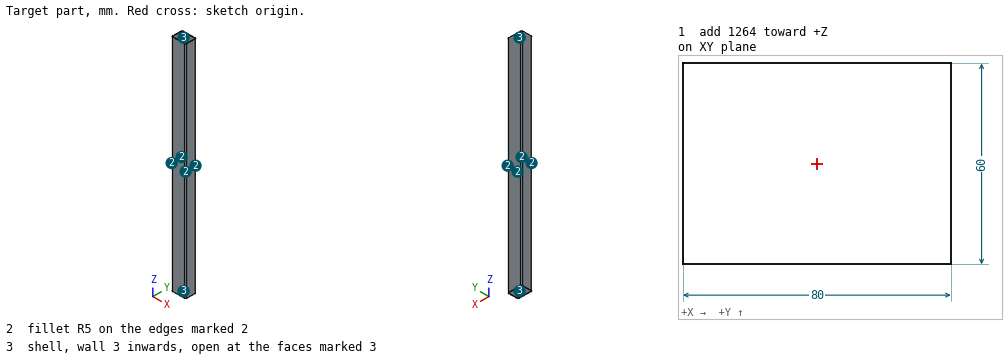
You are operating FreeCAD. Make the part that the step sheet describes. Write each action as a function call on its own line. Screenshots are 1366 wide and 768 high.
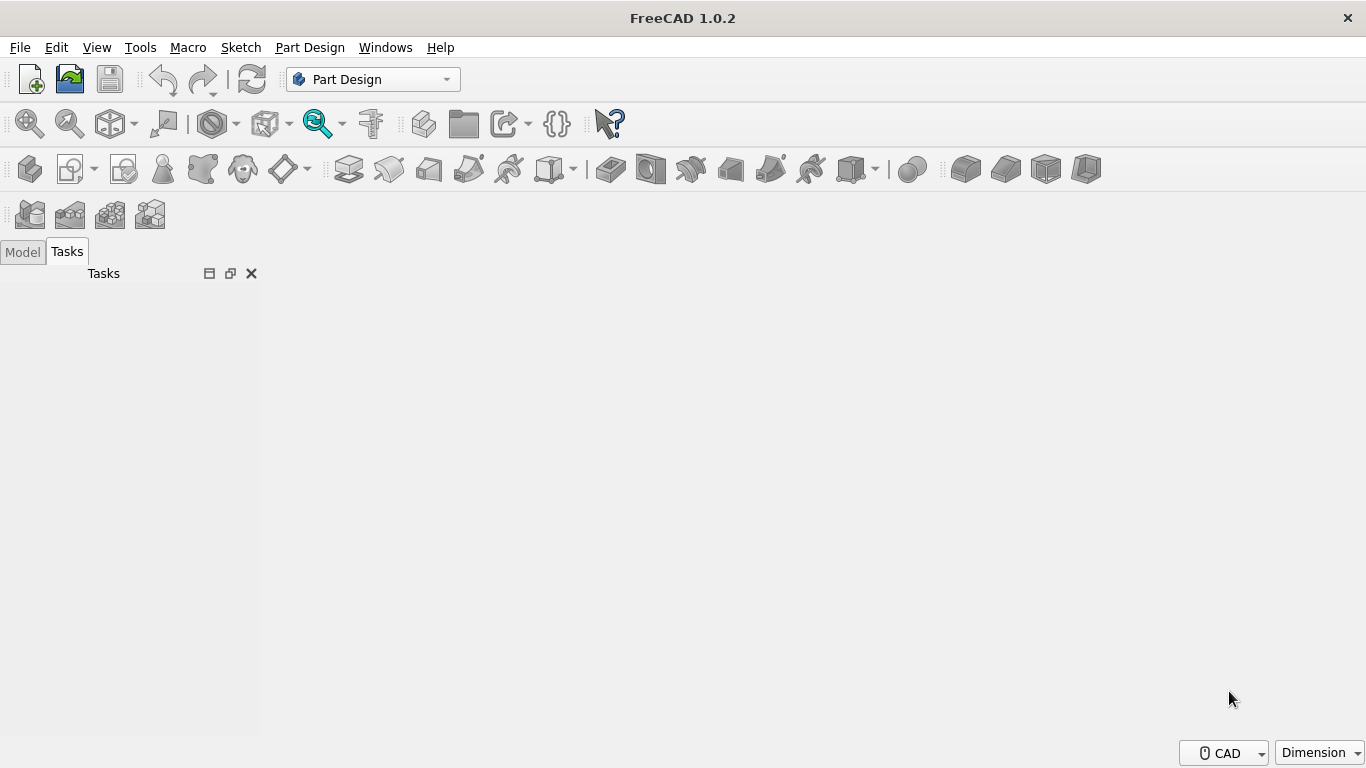
key(ctrl+n)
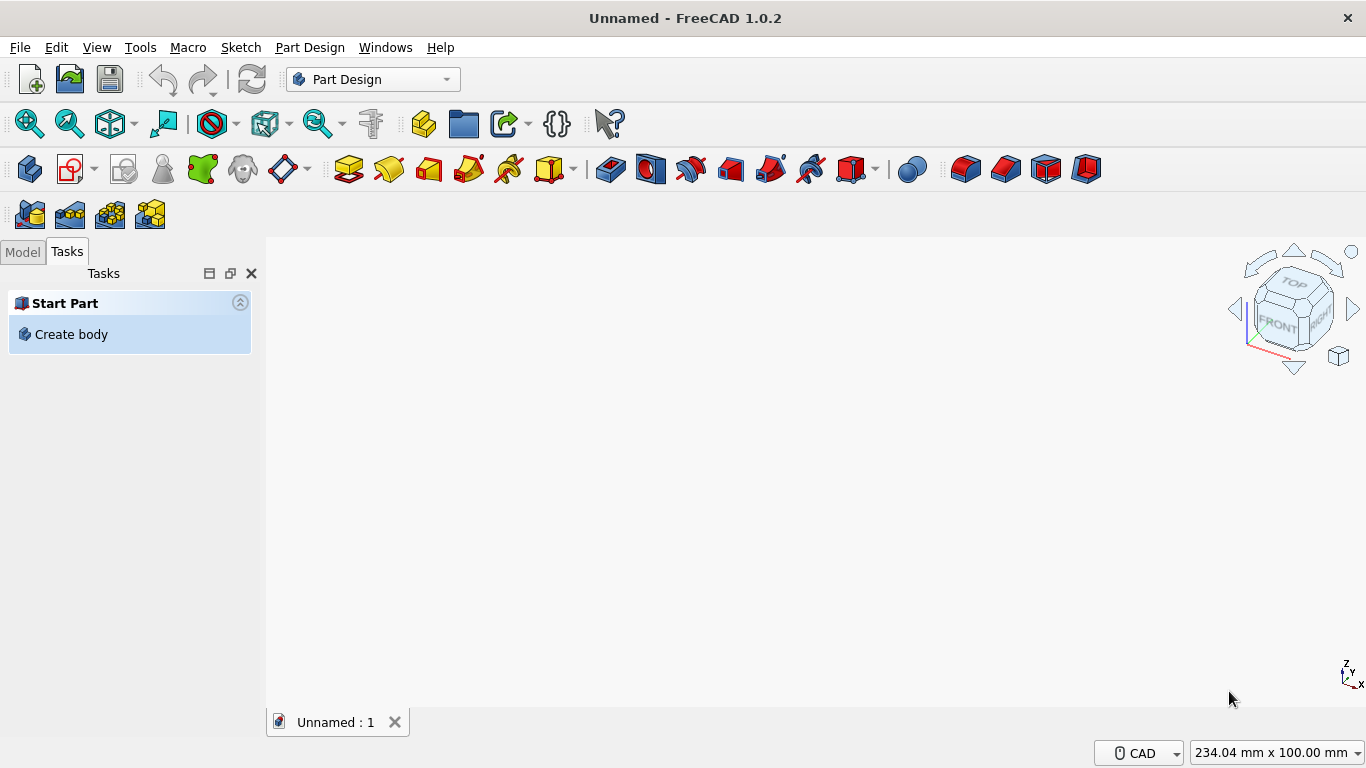
click(70, 170)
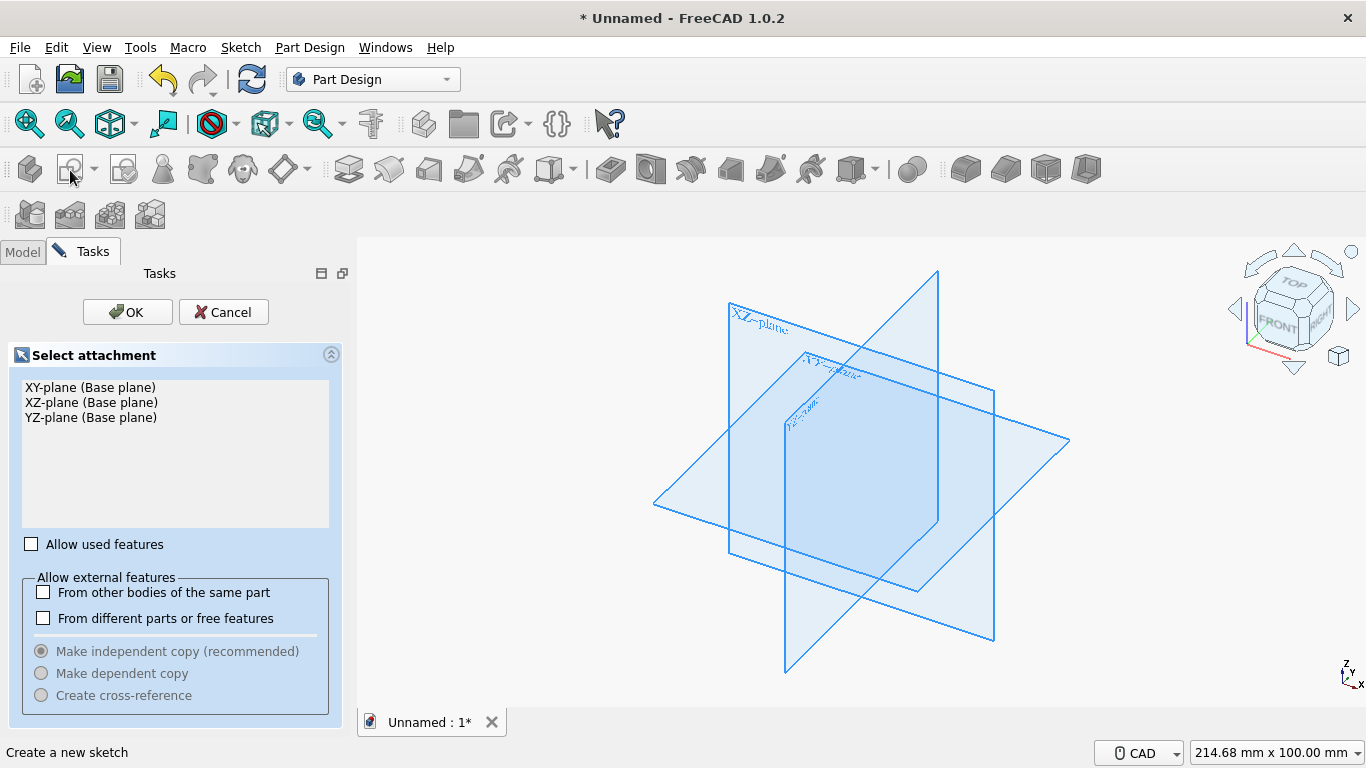
click(82, 388)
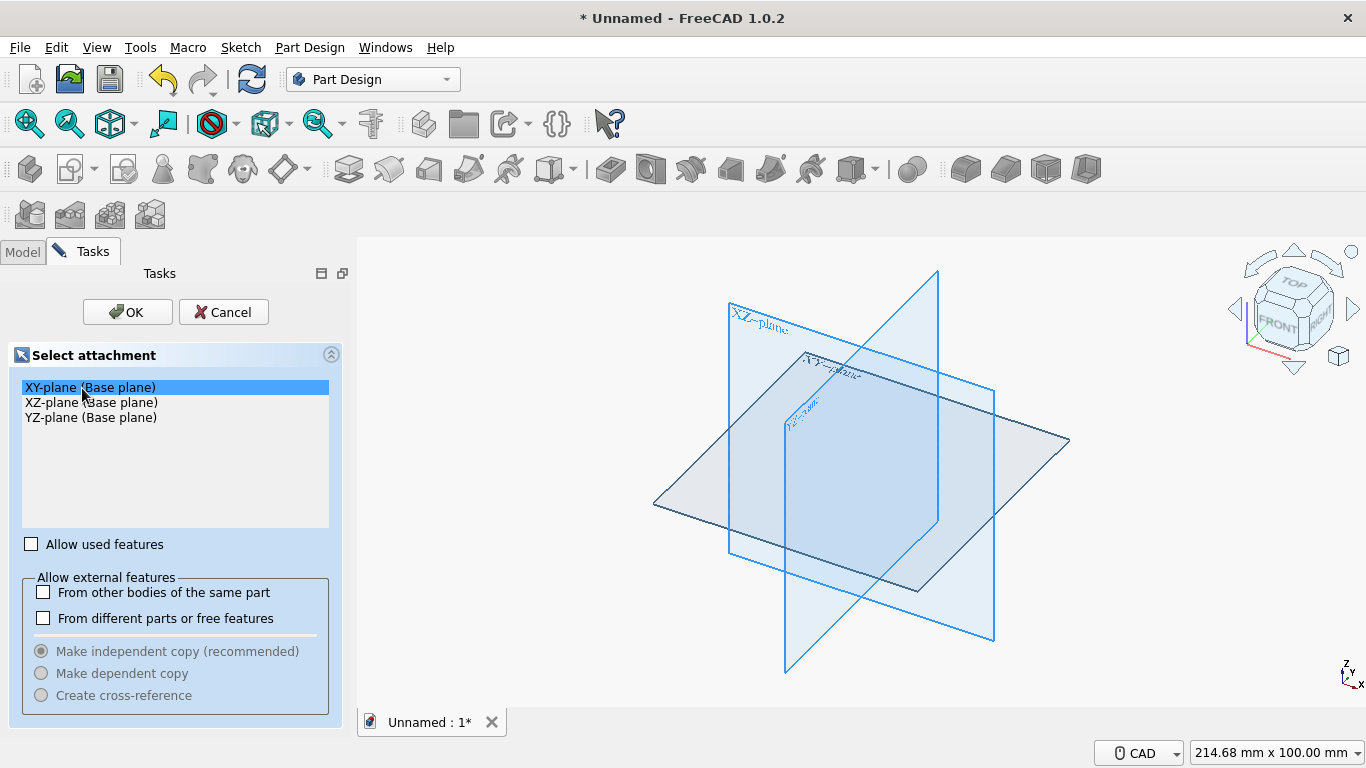
click(128, 312)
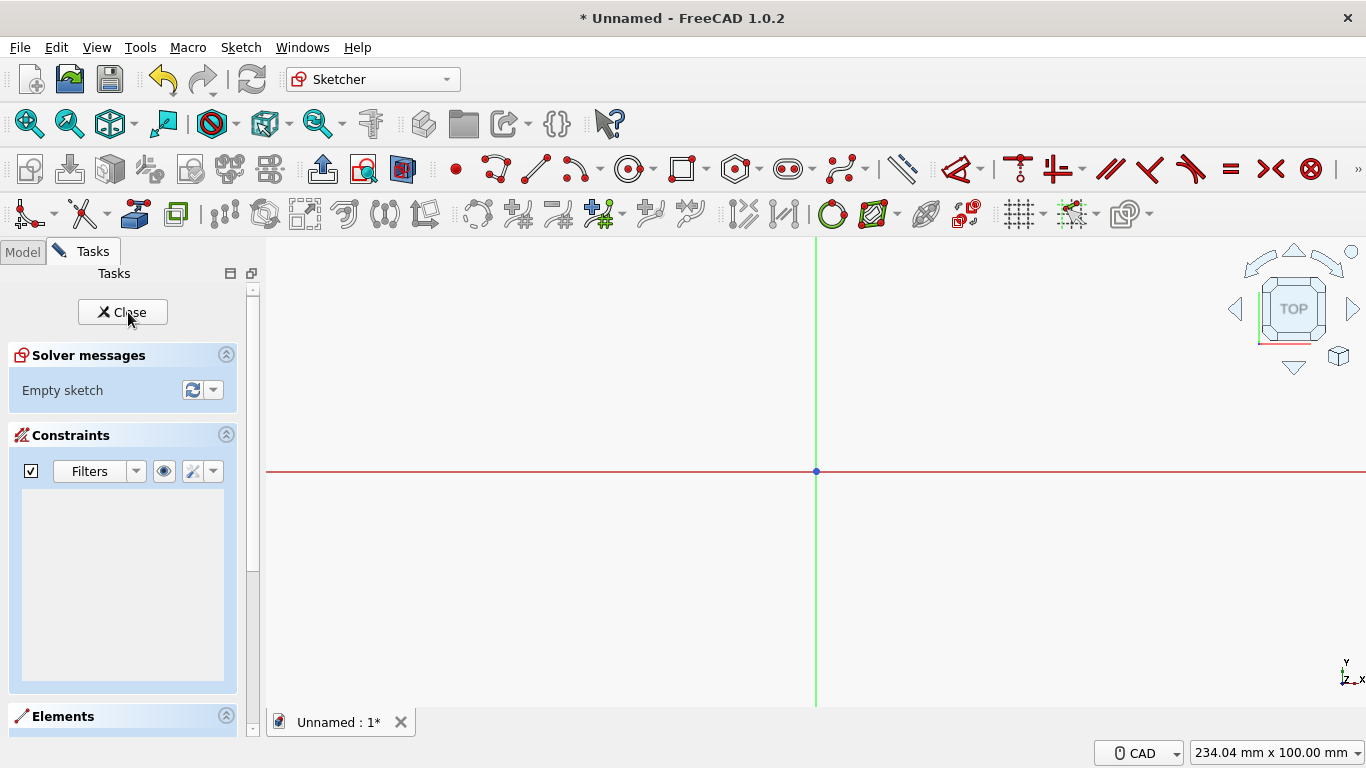
click(708, 170)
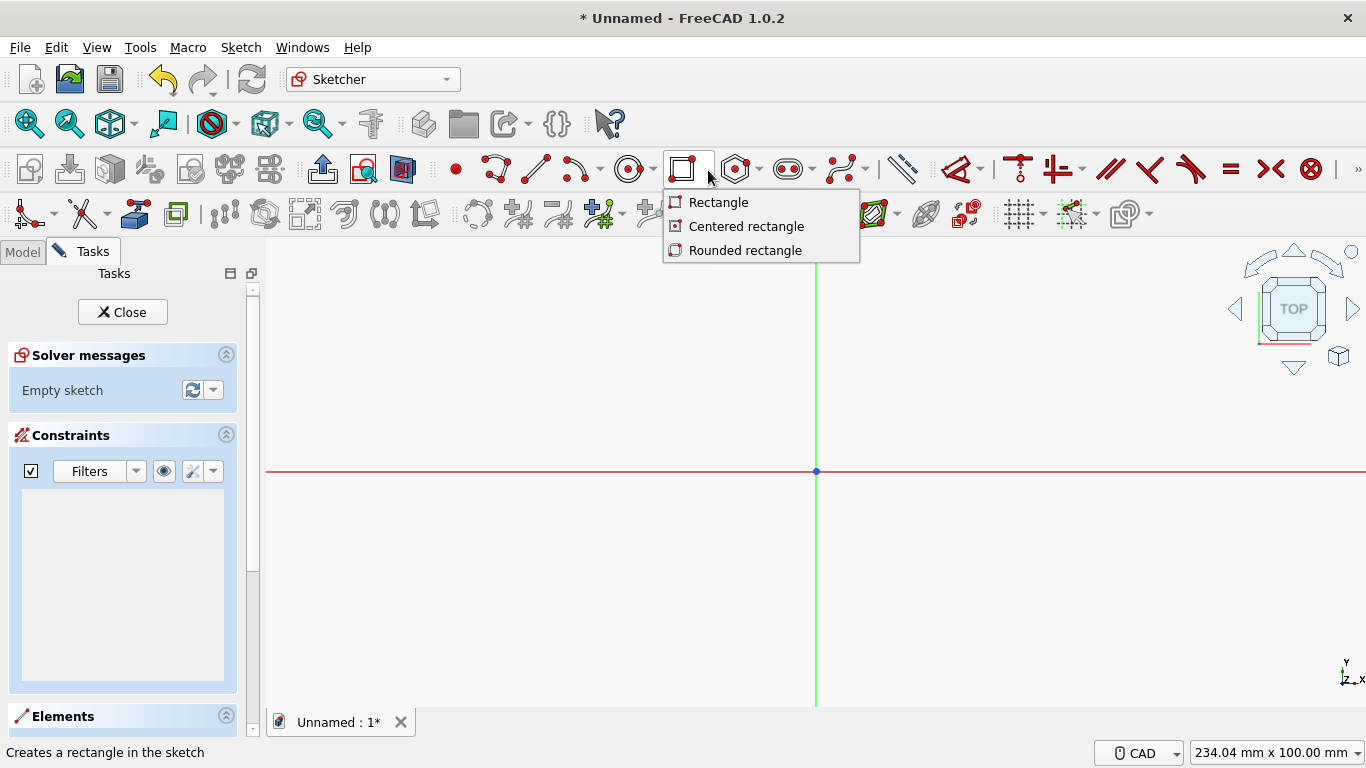
click(762, 226)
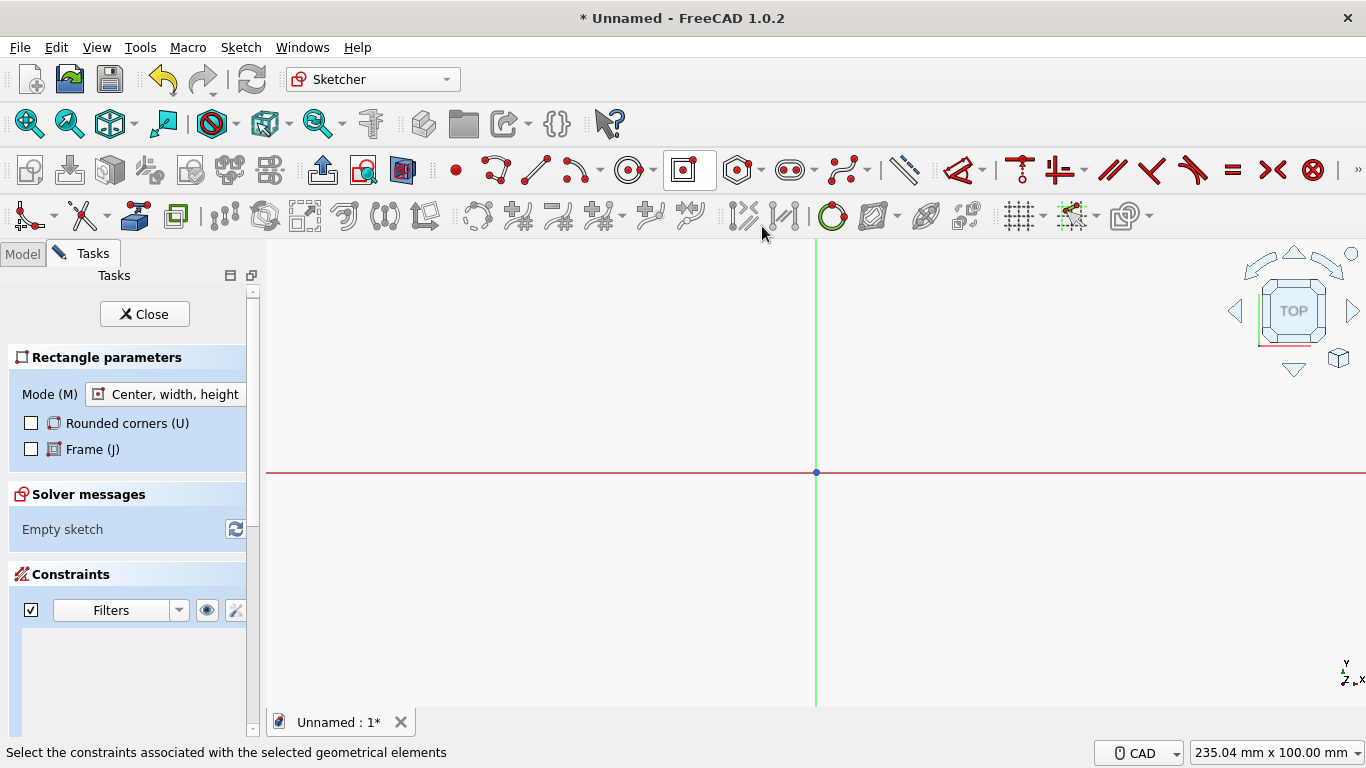
click(816, 473)
move(1003, 333)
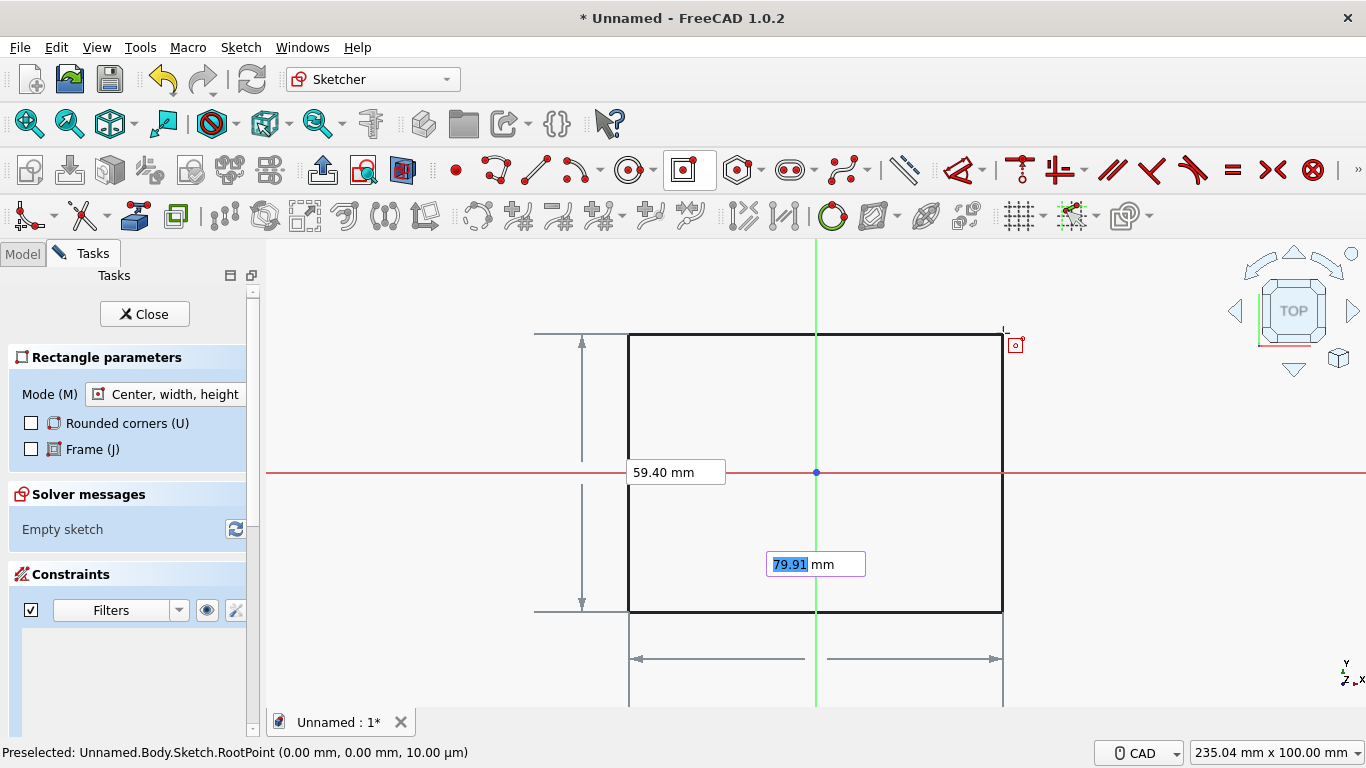
text(80)
key(Tab)
text(60)
key(Return)
key(Escape)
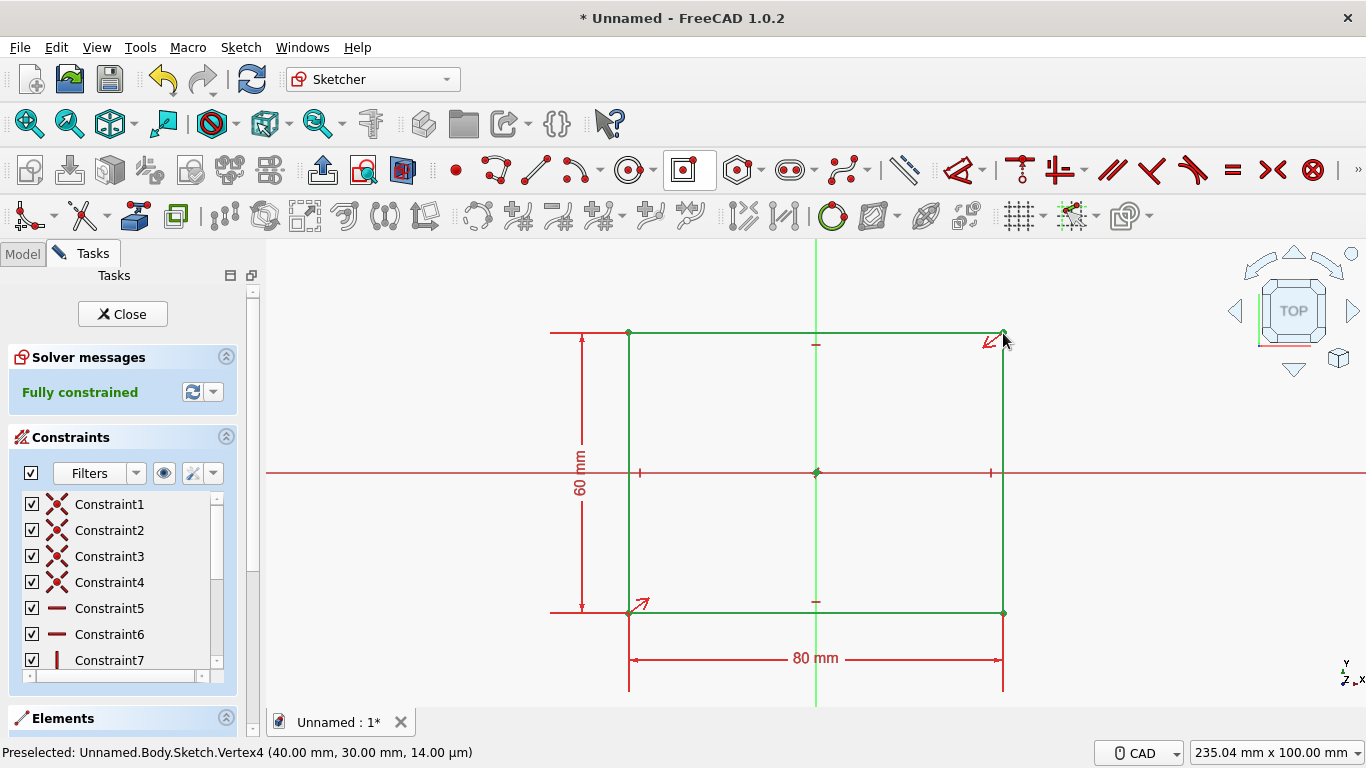
click(123, 314)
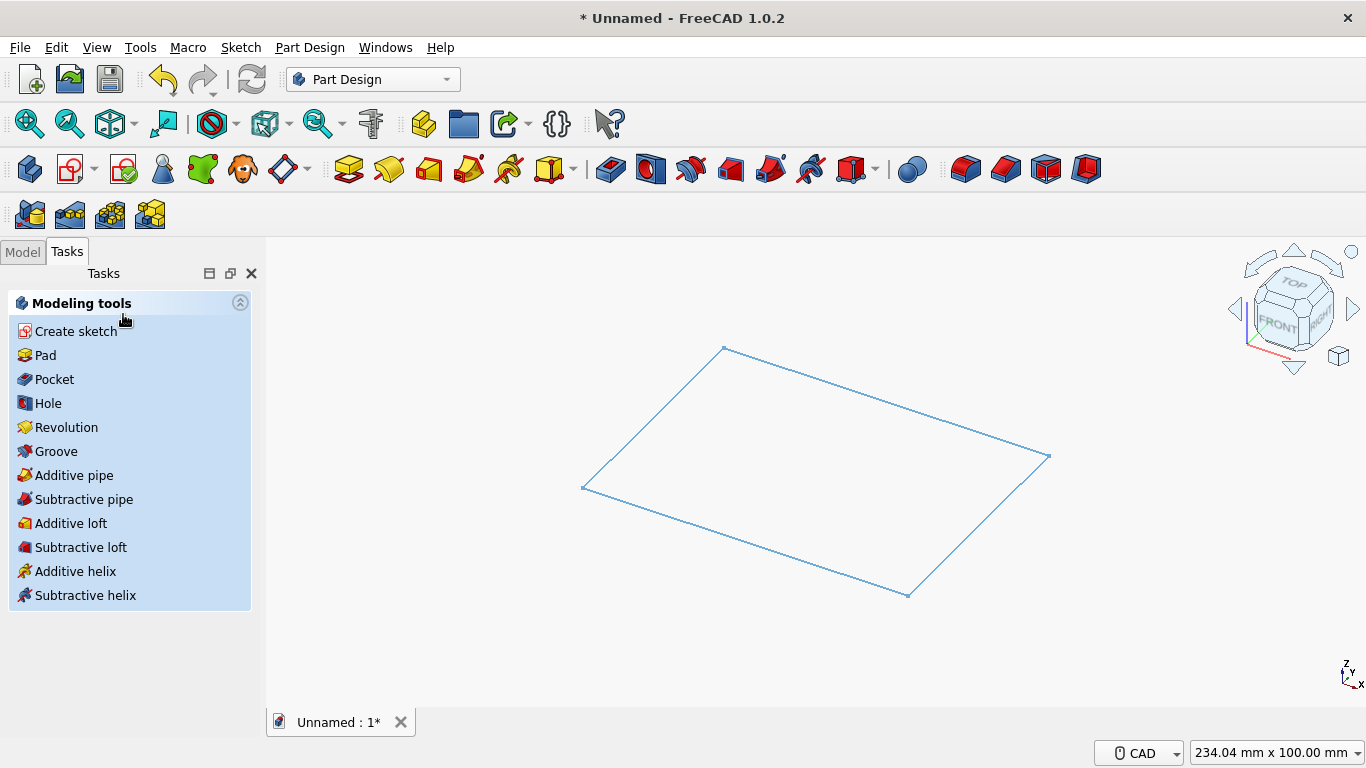
click(350, 170)